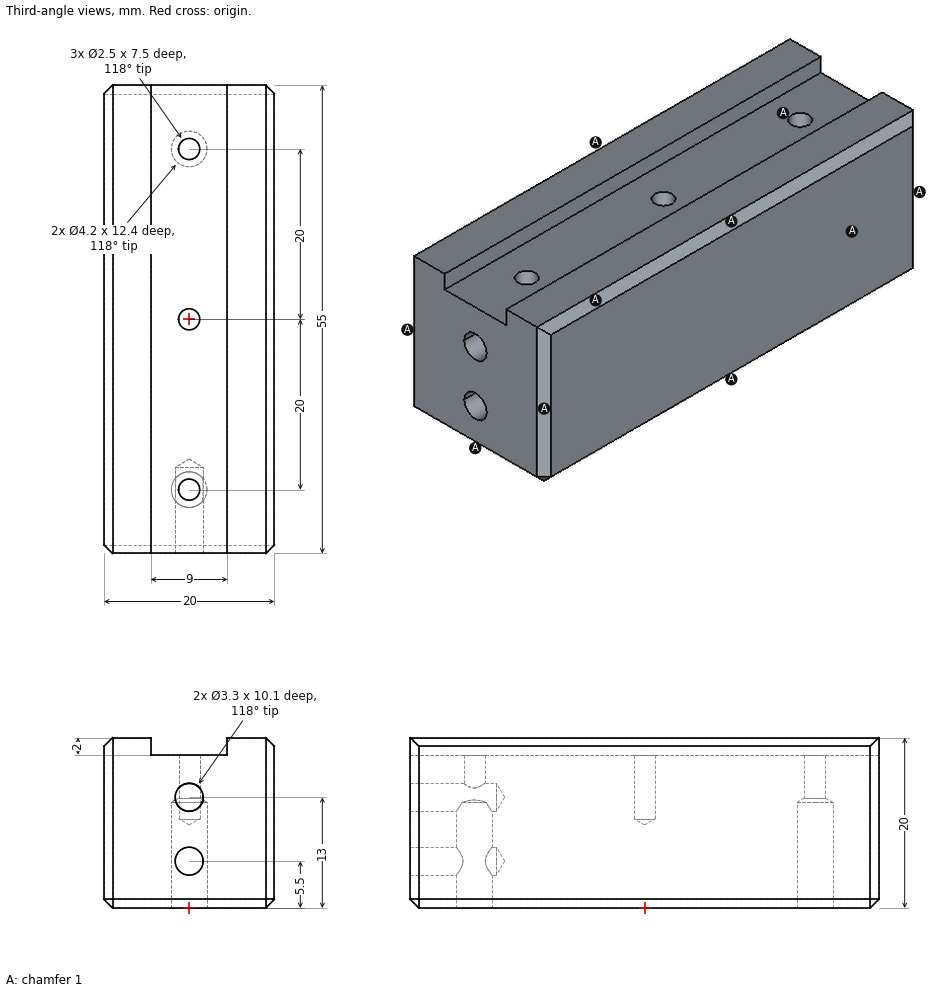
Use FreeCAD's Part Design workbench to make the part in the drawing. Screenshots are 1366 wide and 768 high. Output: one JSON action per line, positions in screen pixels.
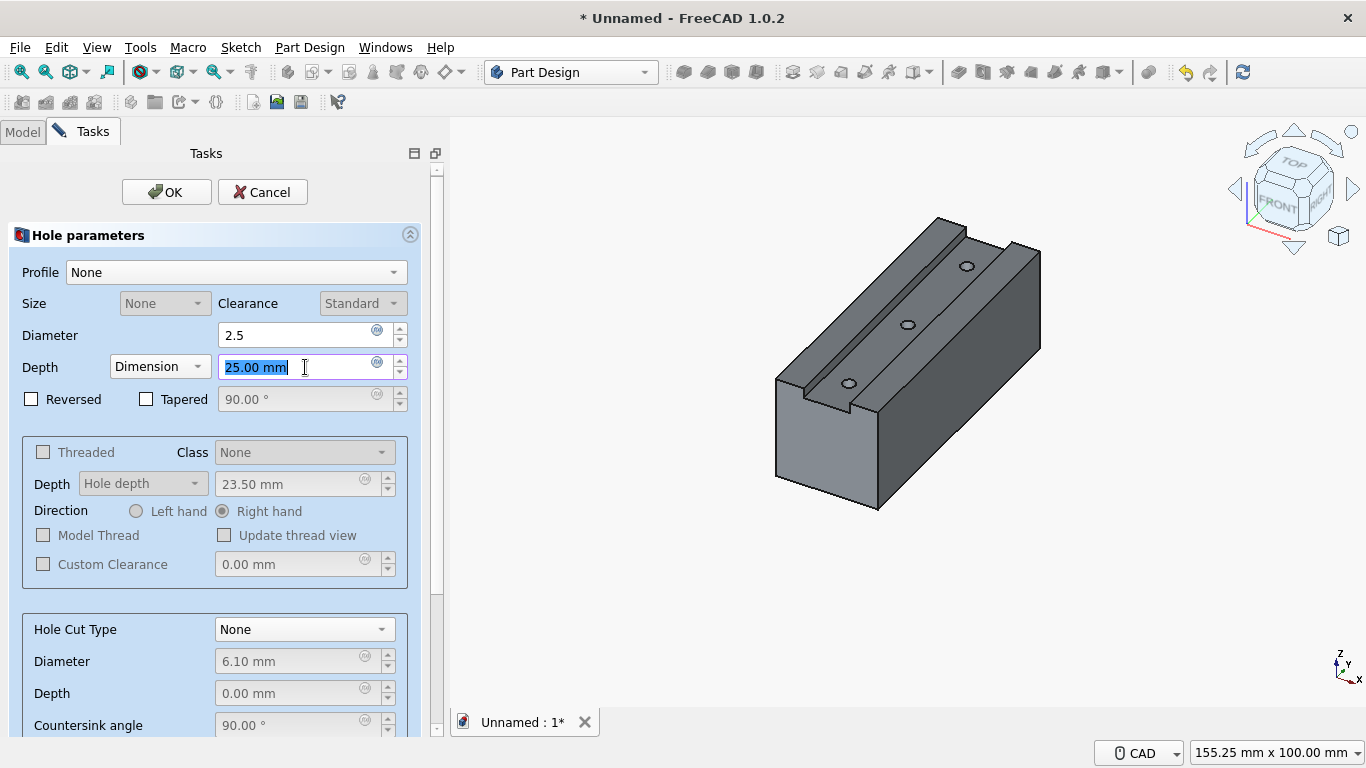
{"action": "type", "text": "7.5"}
{"action": "key", "text": "Tab"}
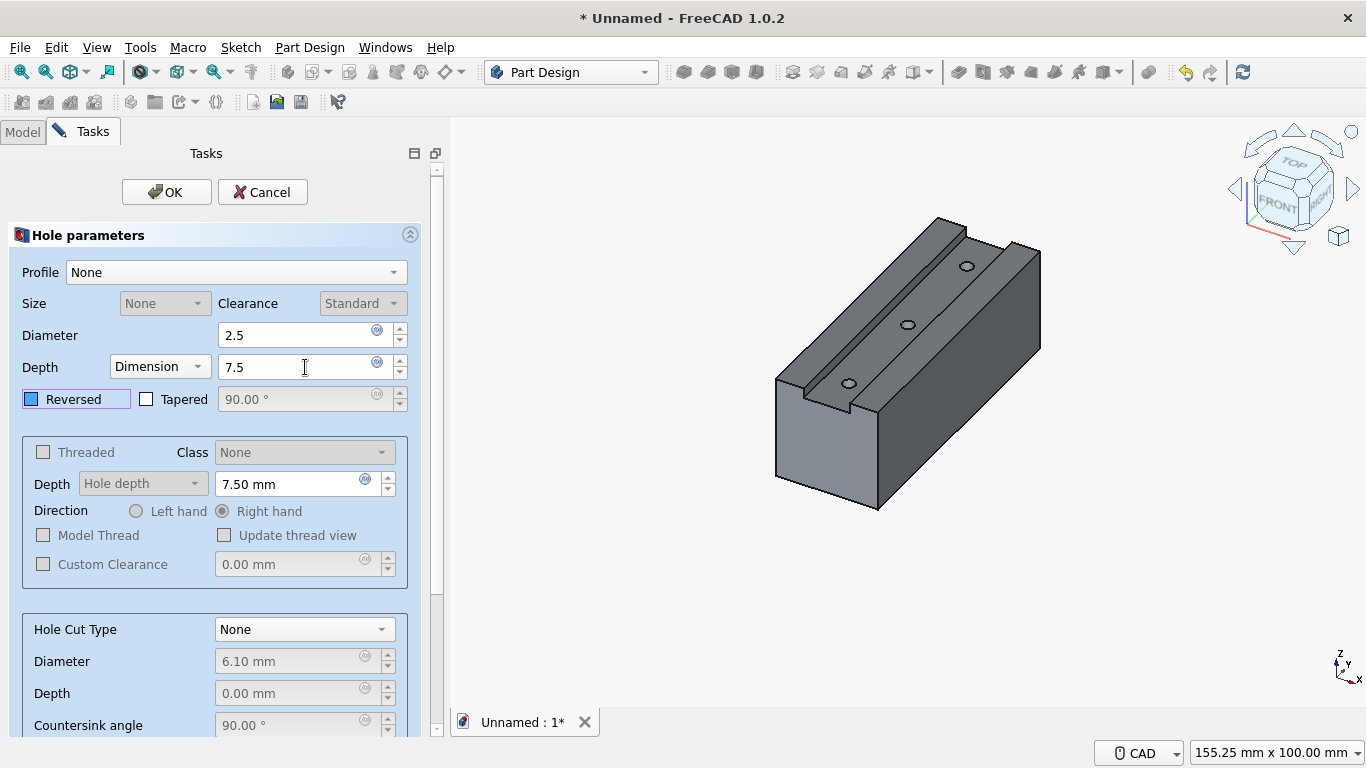
{"action": "left_click", "coordinate": [167, 192]}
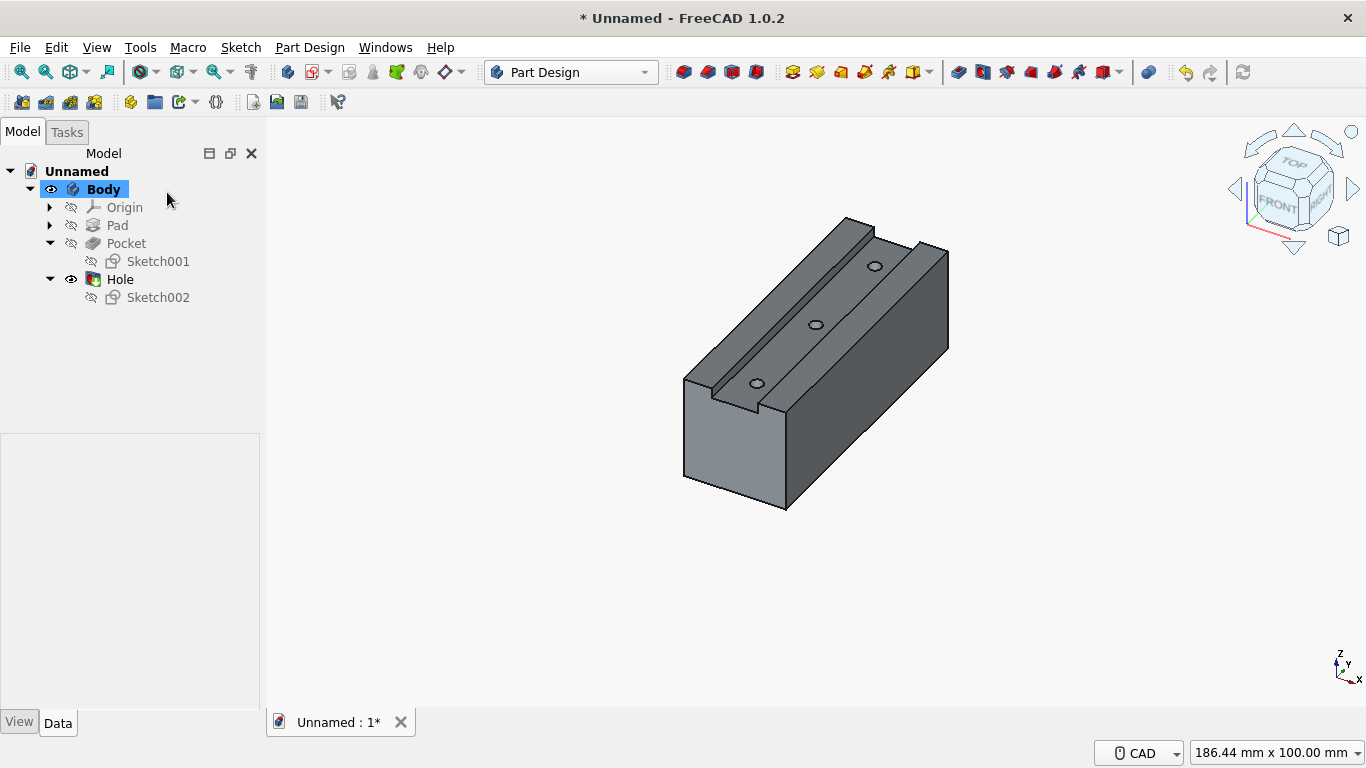
{"action": "left_click", "coordinate": [735, 443]}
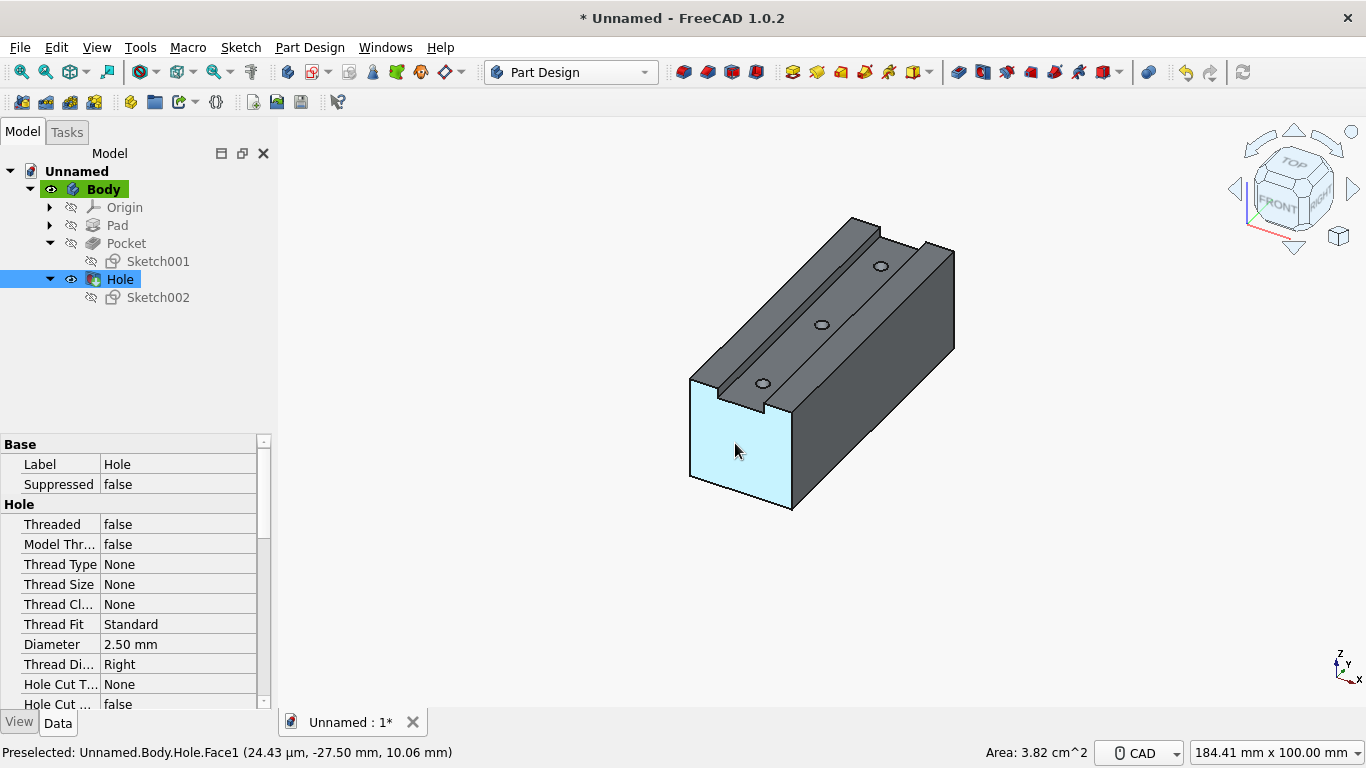
{"action": "left_click", "coordinate": [312, 72]}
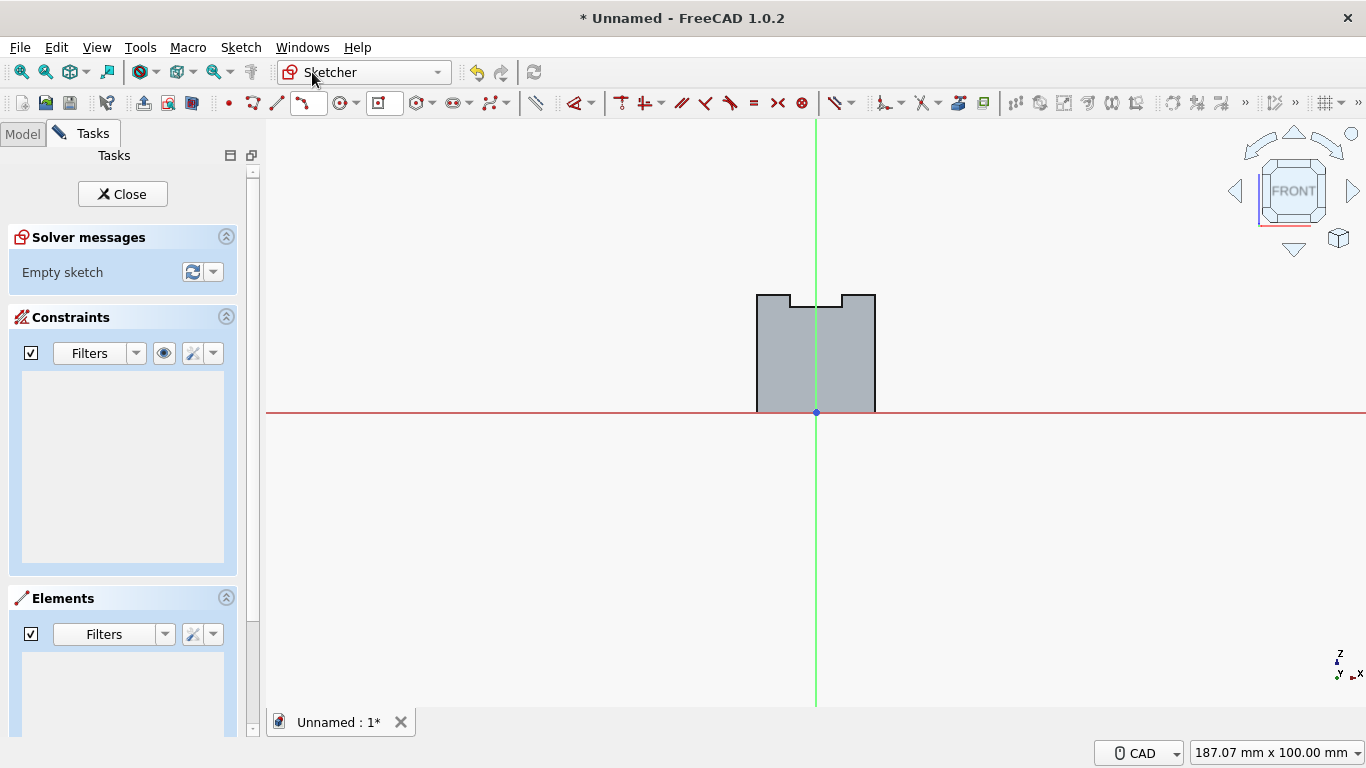
{"action": "scroll", "coordinate": [838, 356], "scroll_direction": "up", "scroll_amount": 7}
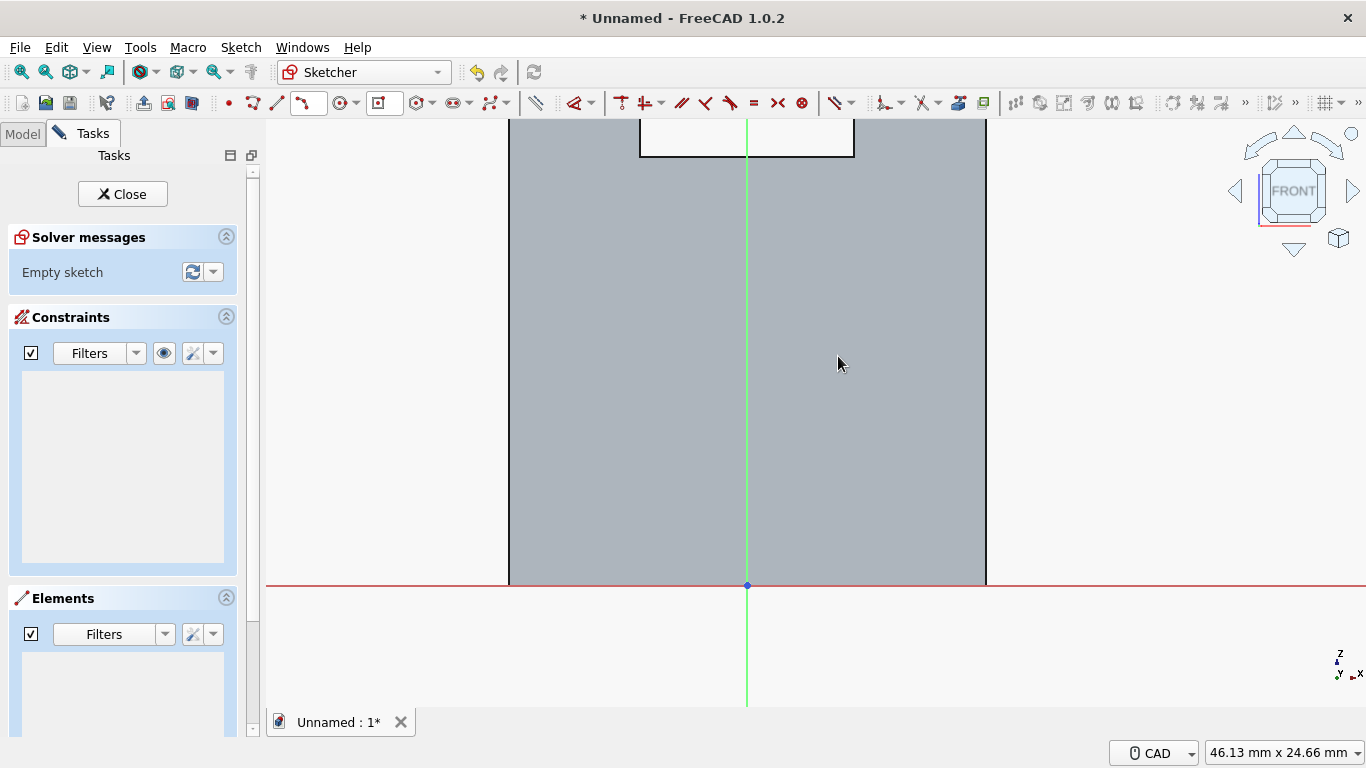
{"action": "left_click", "coordinate": [340, 104]}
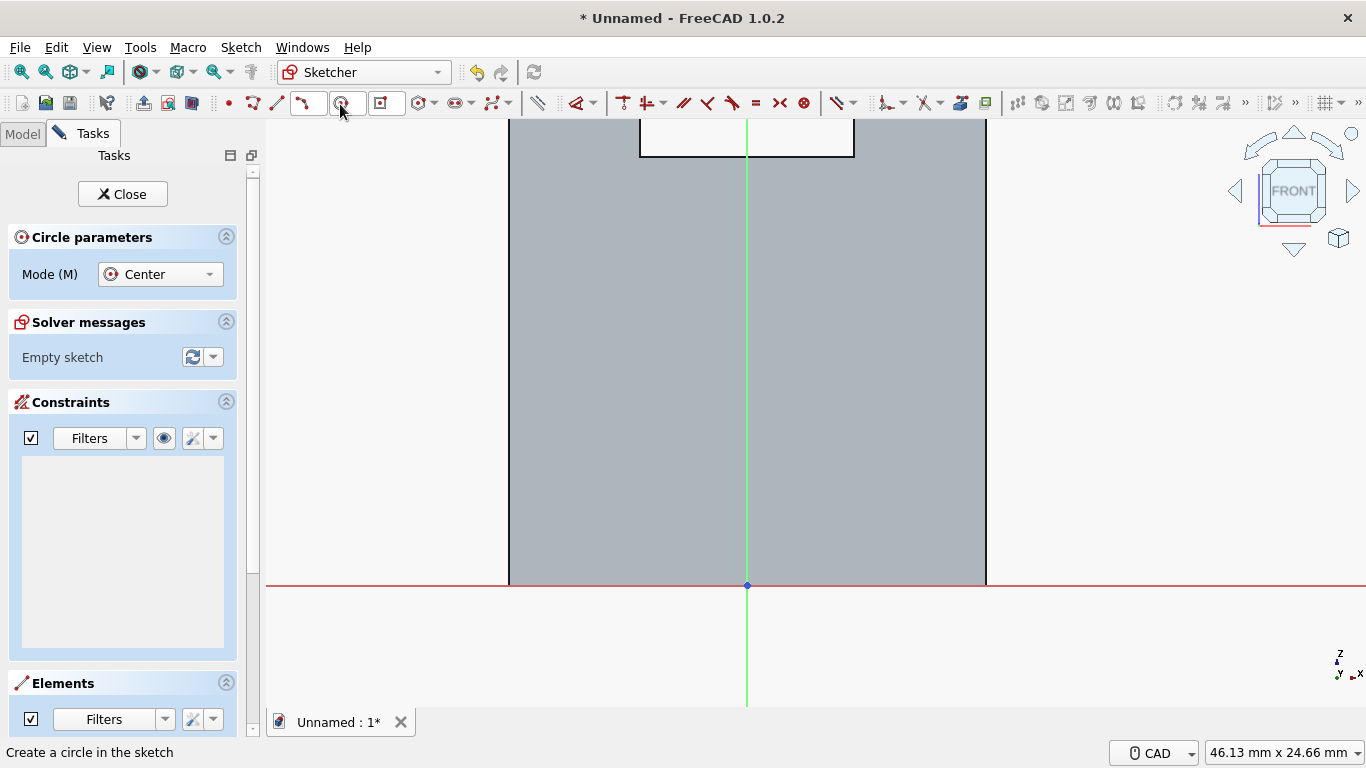
{"action": "left_click", "coordinate": [747, 276]}
{"action": "mouse_move", "coordinate": [775, 248]}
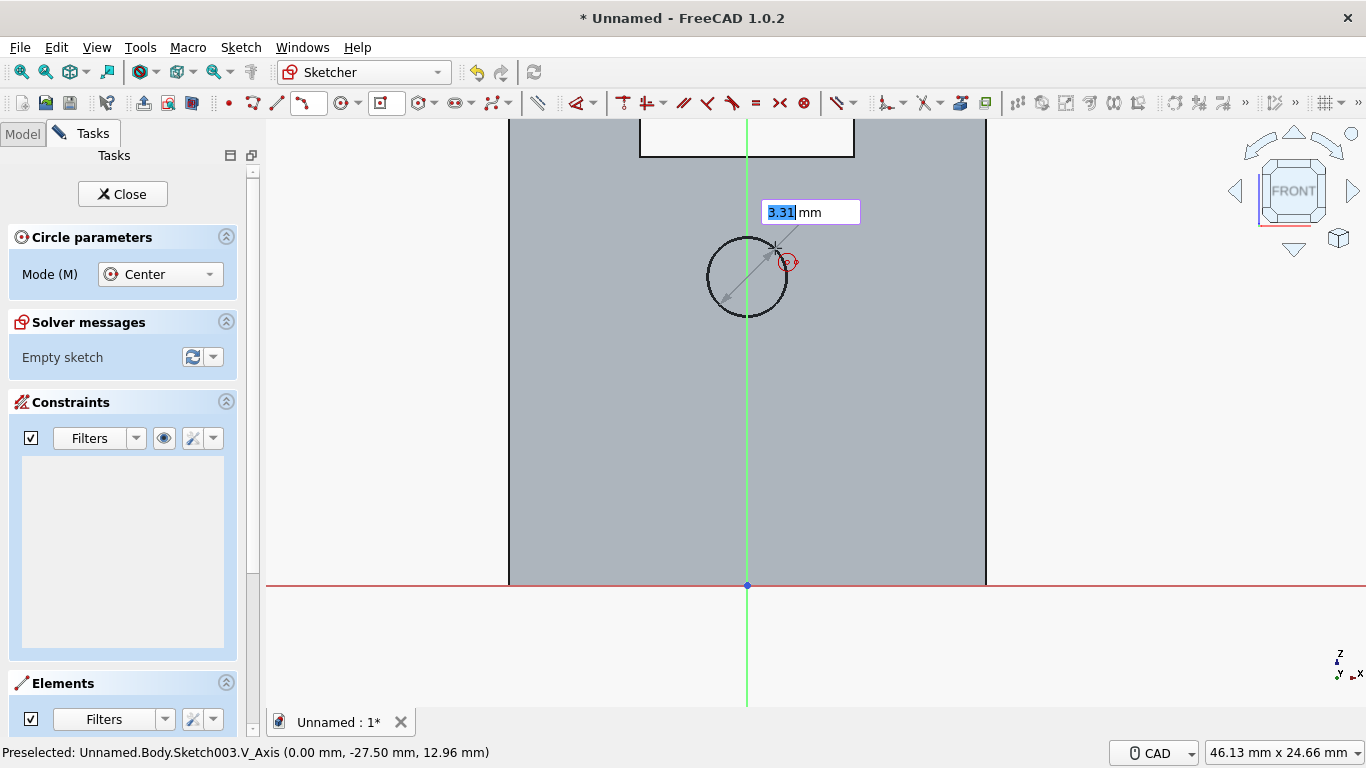
{"action": "type", "text": "3.3"}
{"action": "key", "text": "Return"}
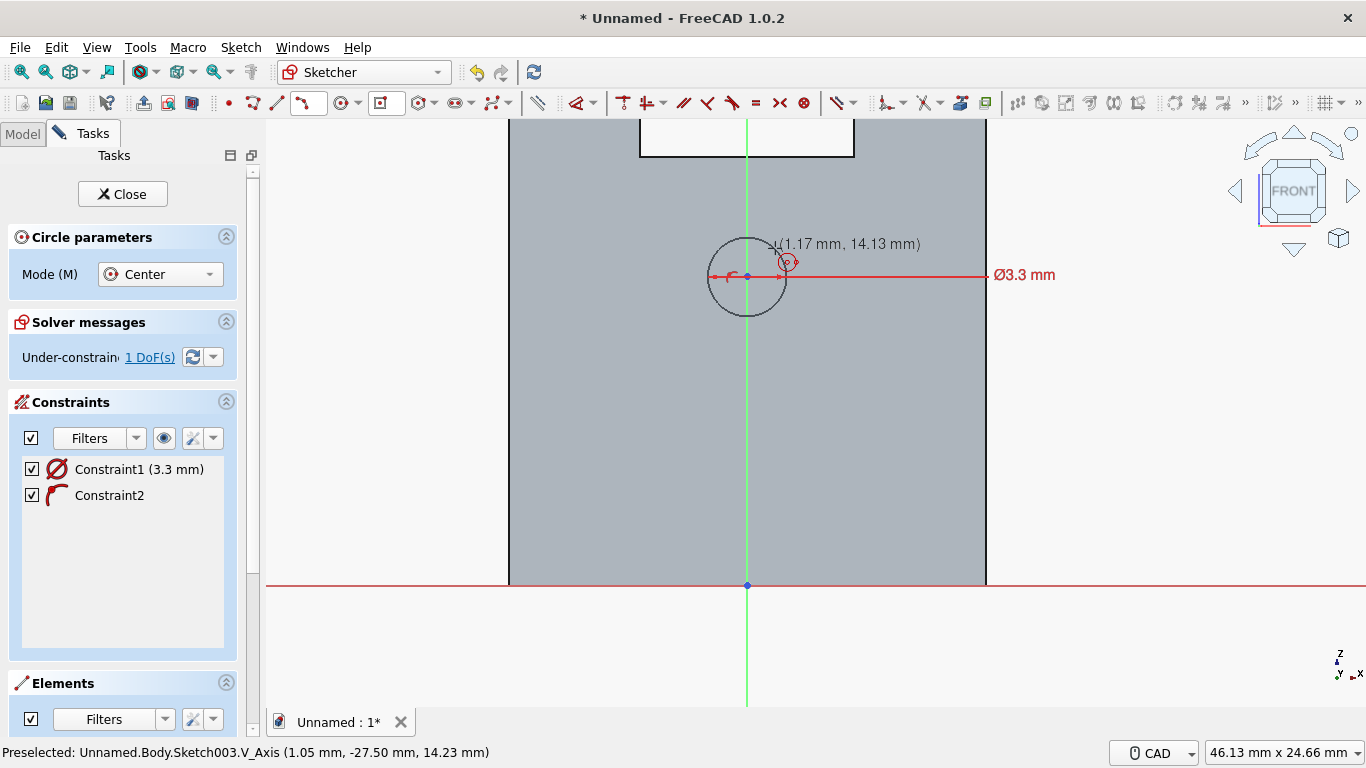
{"action": "left_click", "coordinate": [747, 455]}
{"action": "mouse_move", "coordinate": [775, 427]}